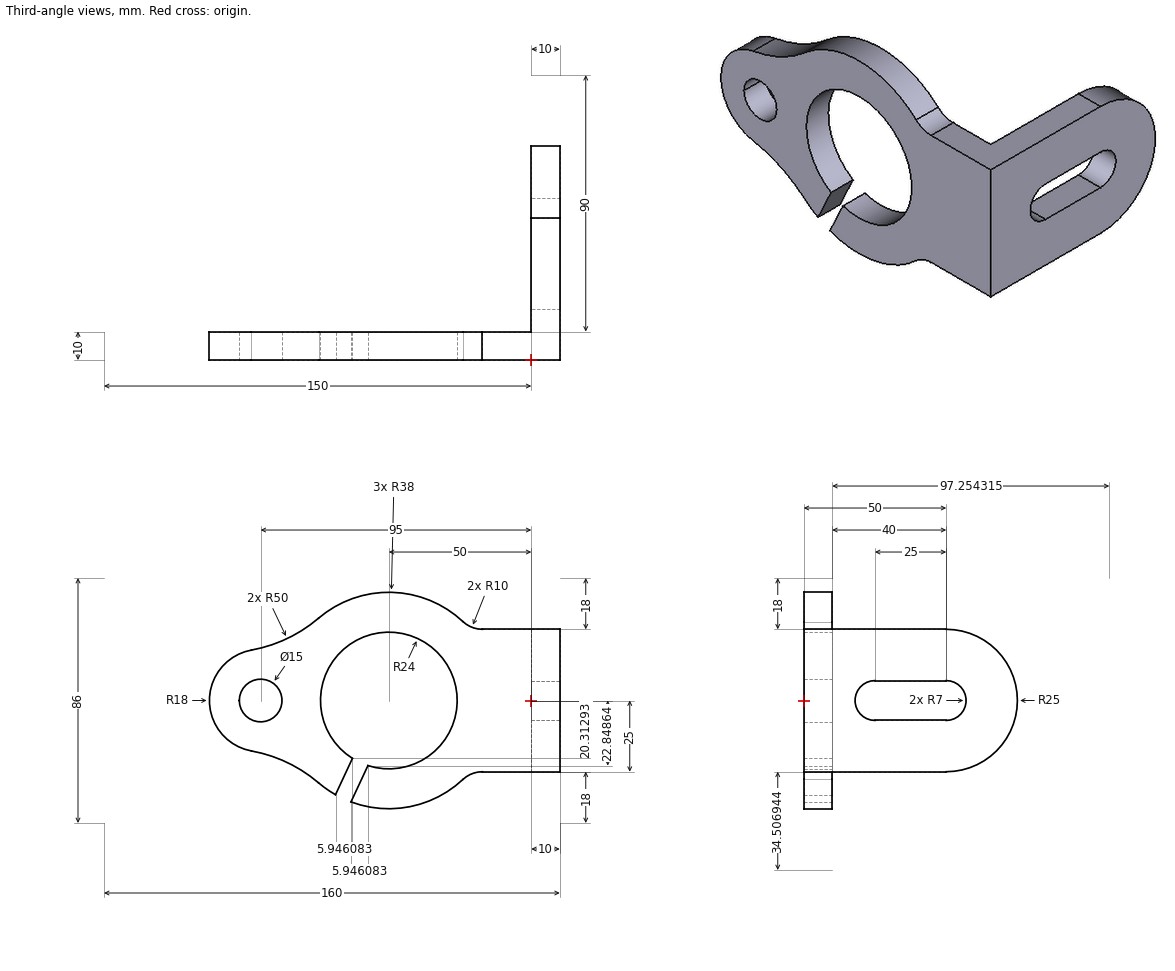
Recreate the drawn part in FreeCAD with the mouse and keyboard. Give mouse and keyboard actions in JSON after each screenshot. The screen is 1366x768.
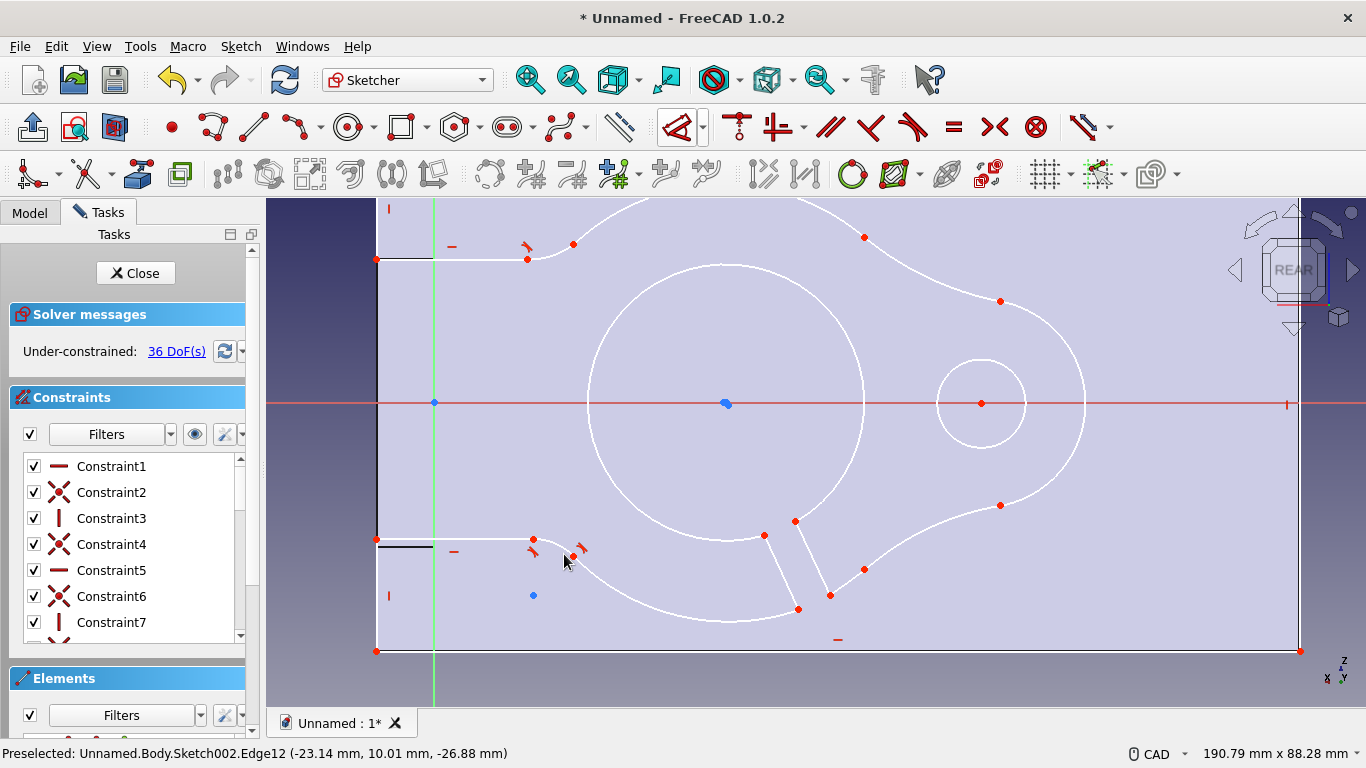
{"action": "left_click", "coordinate": [542, 258]}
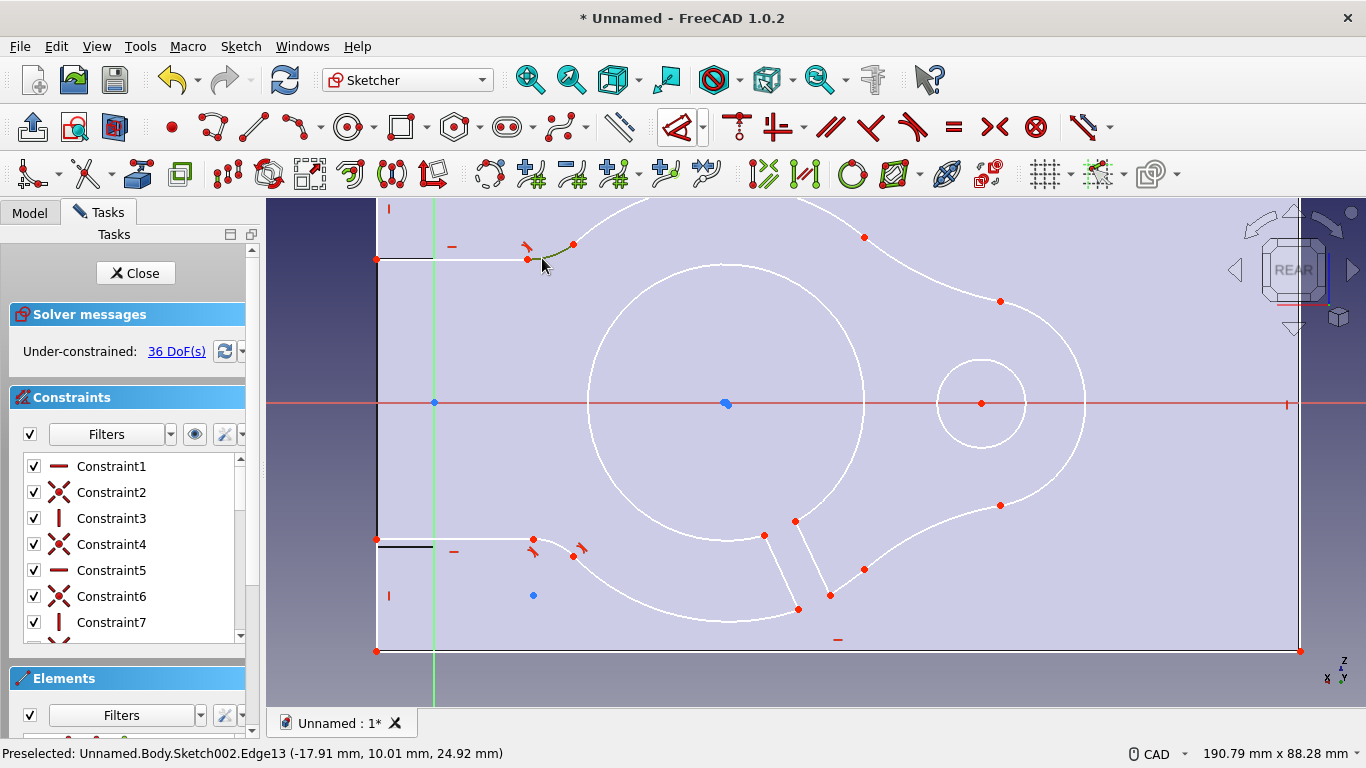
{"action": "scroll", "coordinate": [563, 554], "scroll_direction": "down", "scroll_amount": 2}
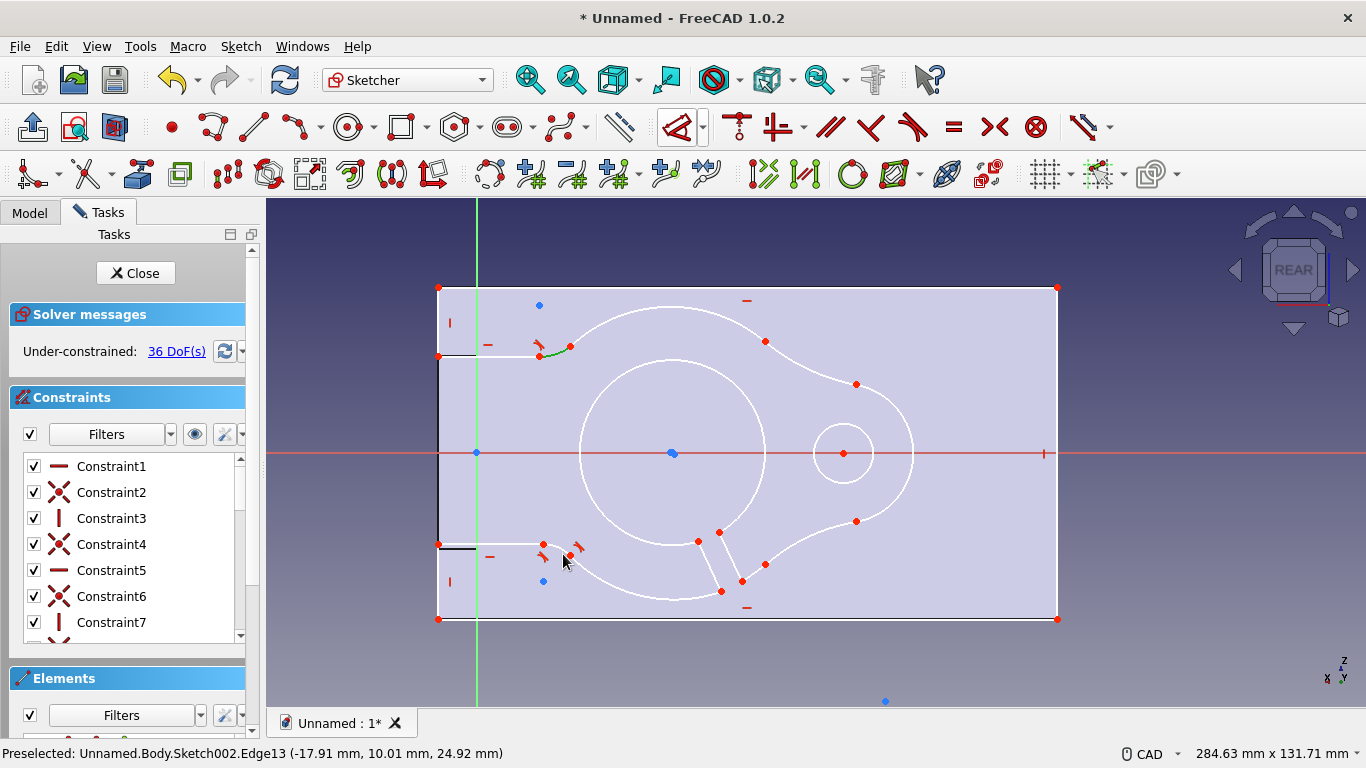
{"action": "left_click", "coordinate": [709, 312]}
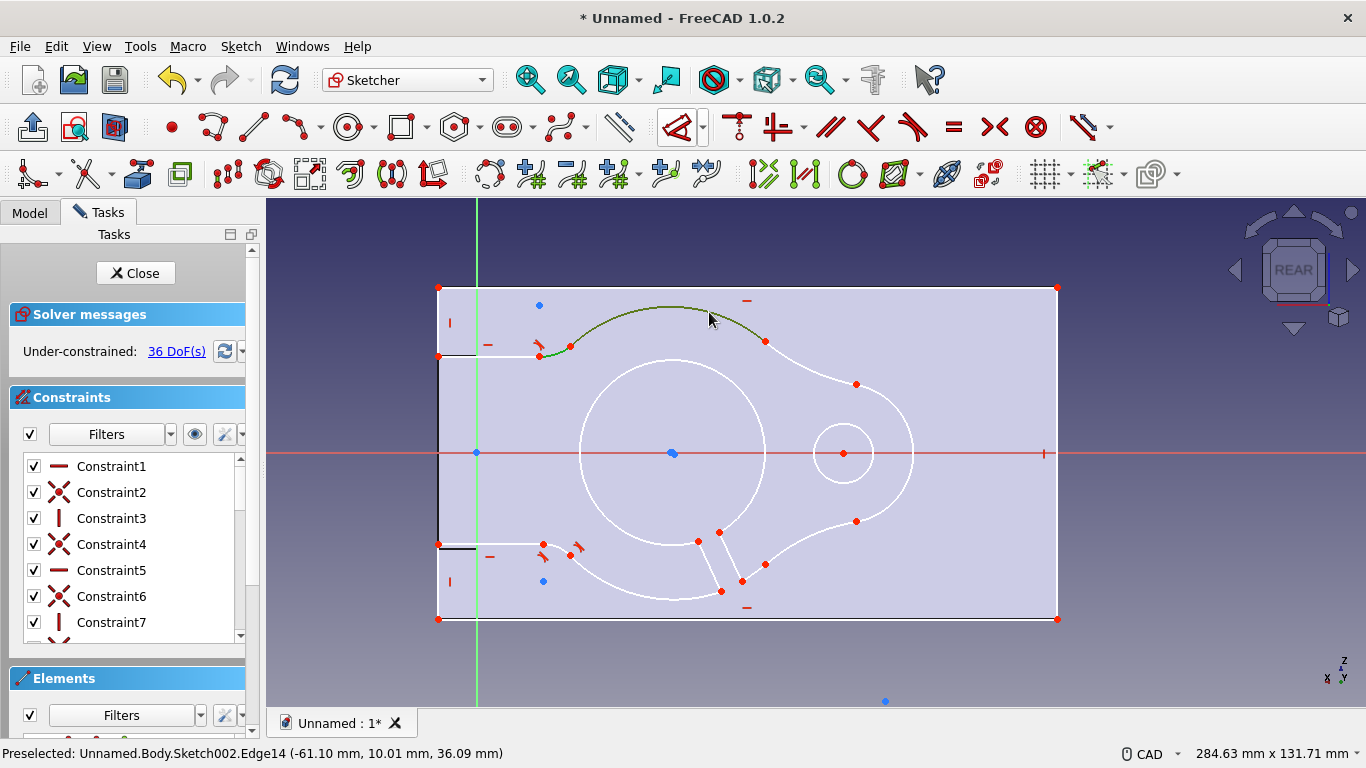
{"action": "left_click", "coordinate": [913, 128]}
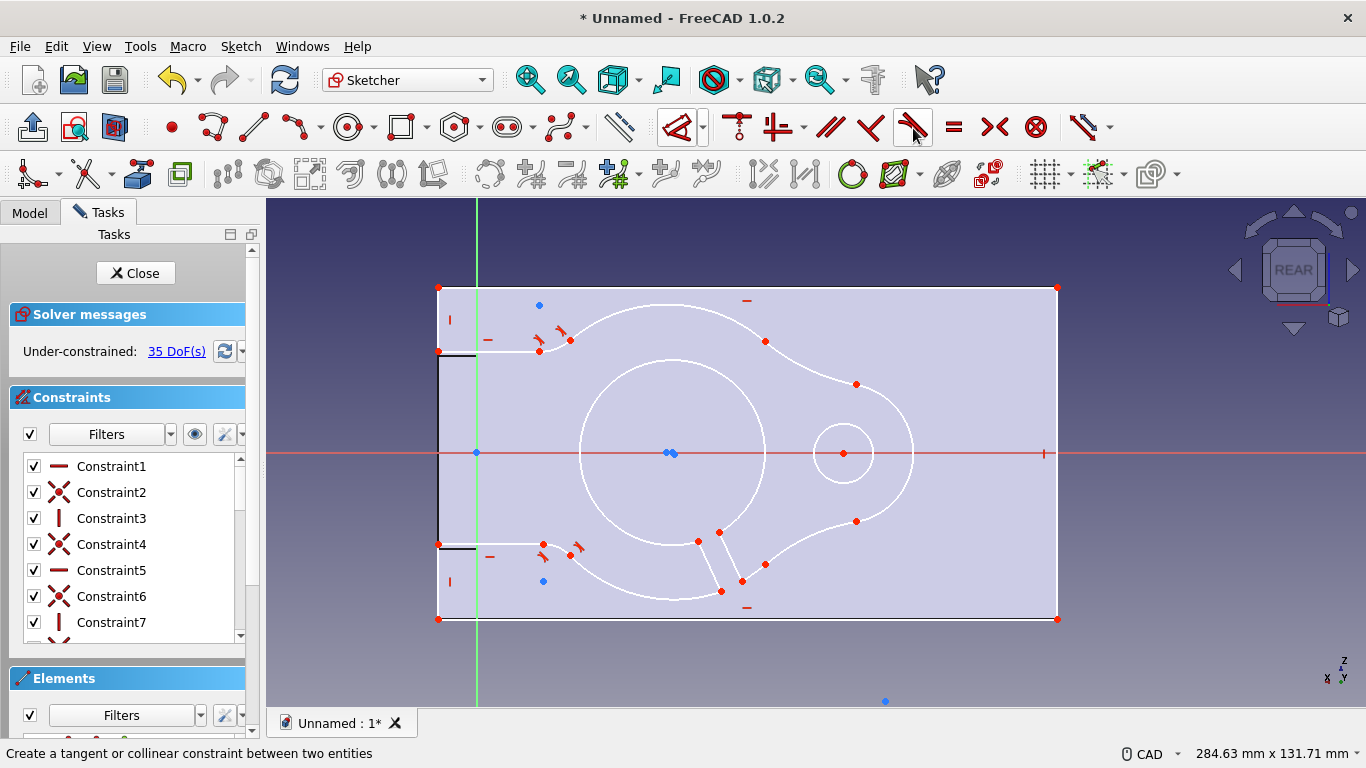
{"action": "left_click", "coordinate": [710, 311]}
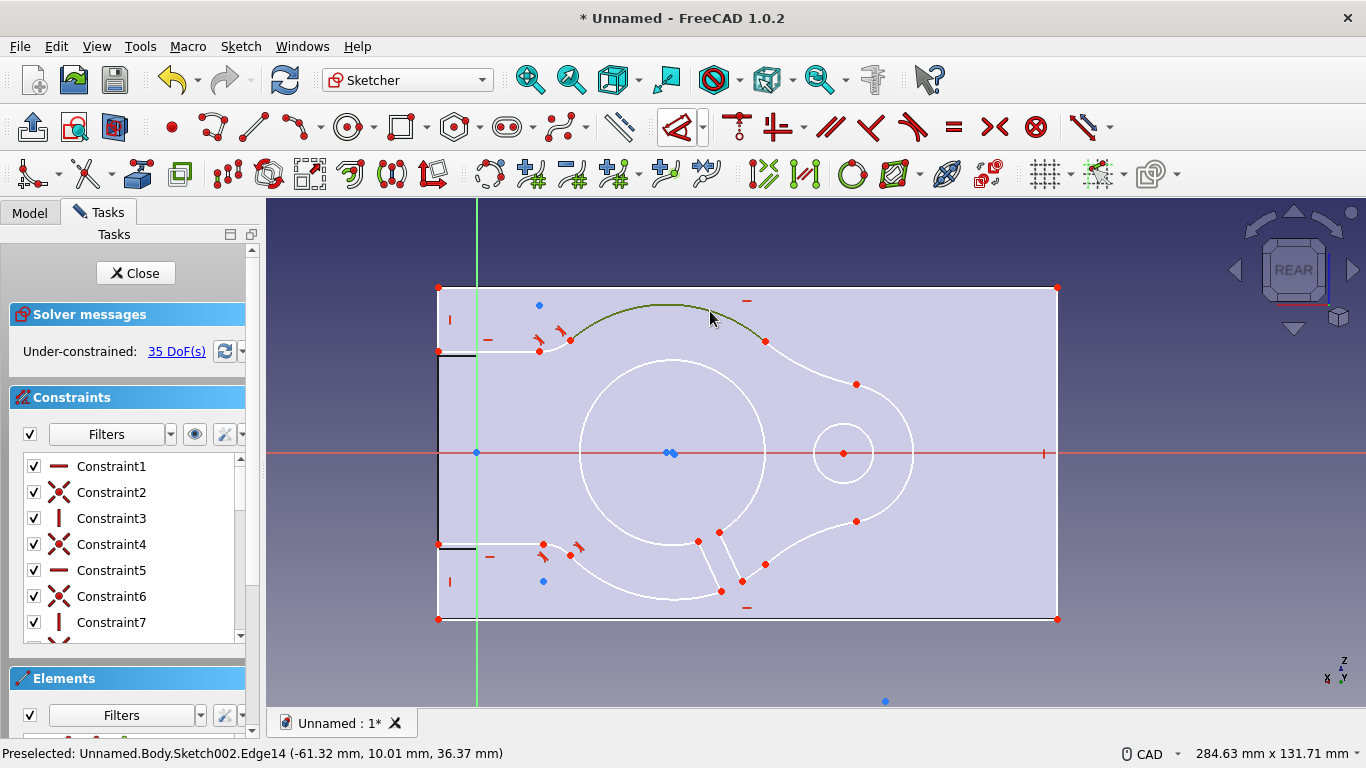
{"action": "left_click", "coordinate": [790, 359]}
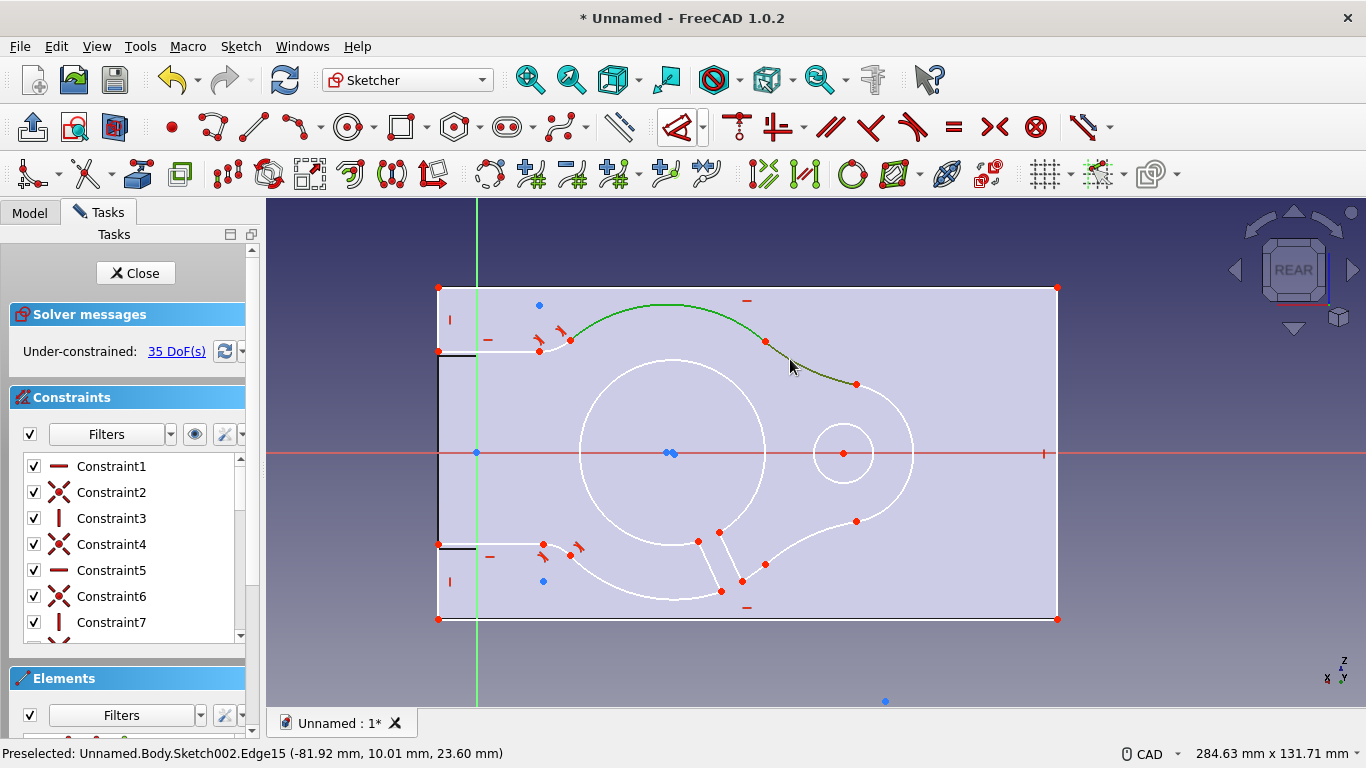
{"action": "key", "text": "t"}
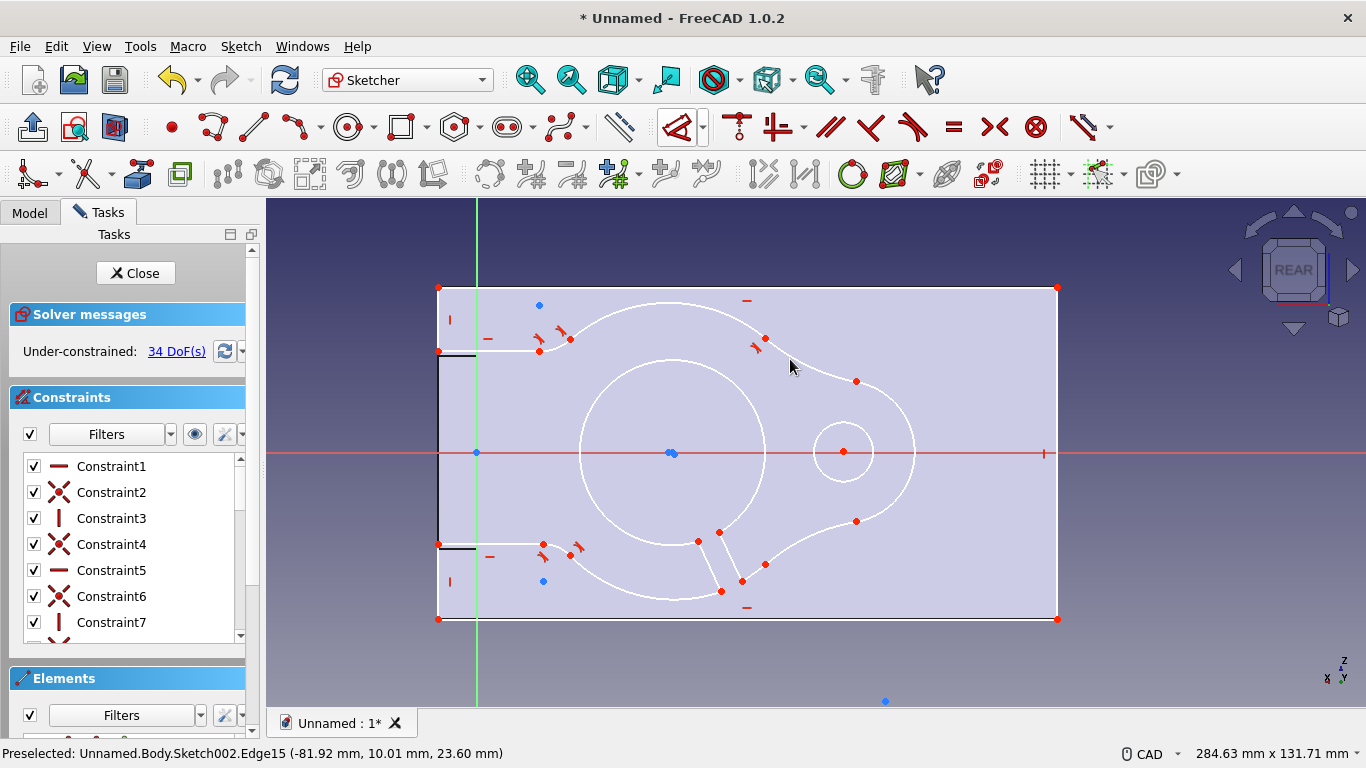
{"action": "left_click", "coordinate": [790, 356]}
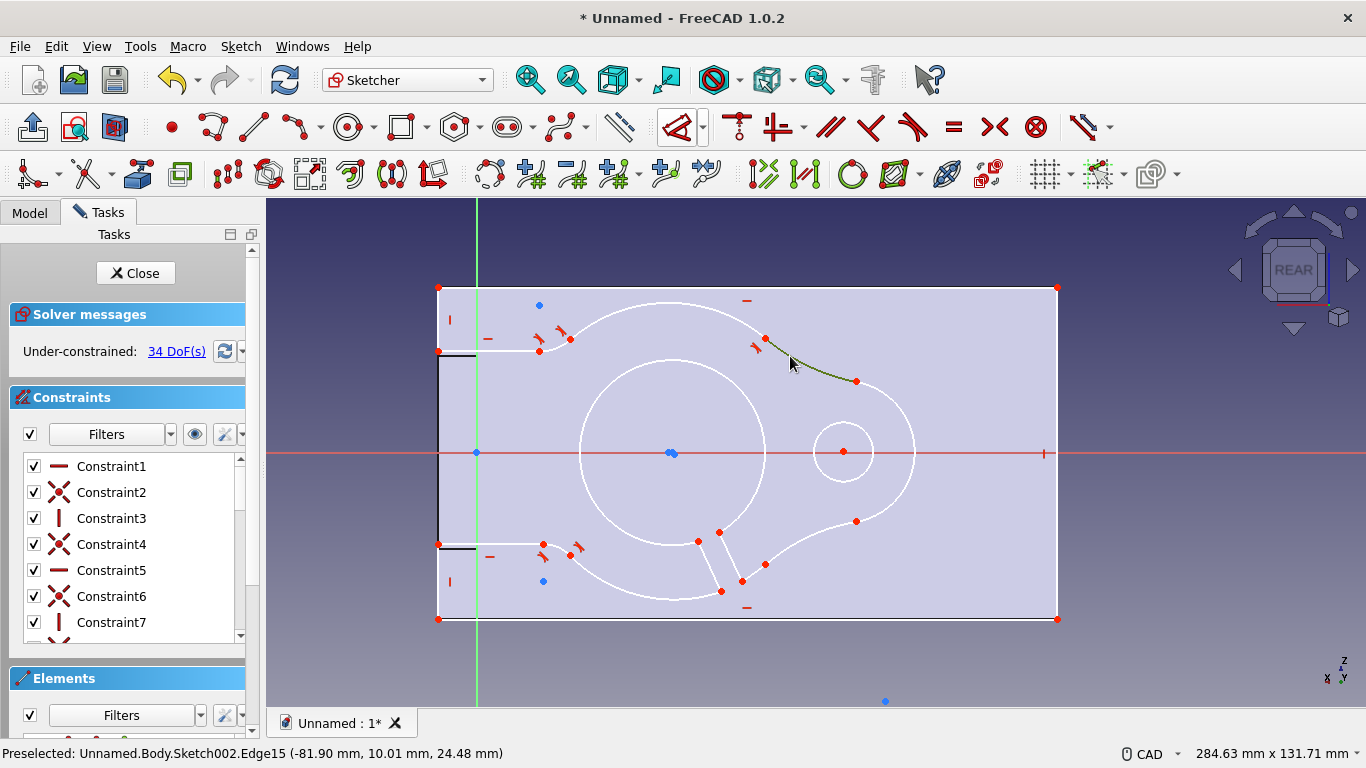
{"action": "left_click", "coordinate": [904, 489]}